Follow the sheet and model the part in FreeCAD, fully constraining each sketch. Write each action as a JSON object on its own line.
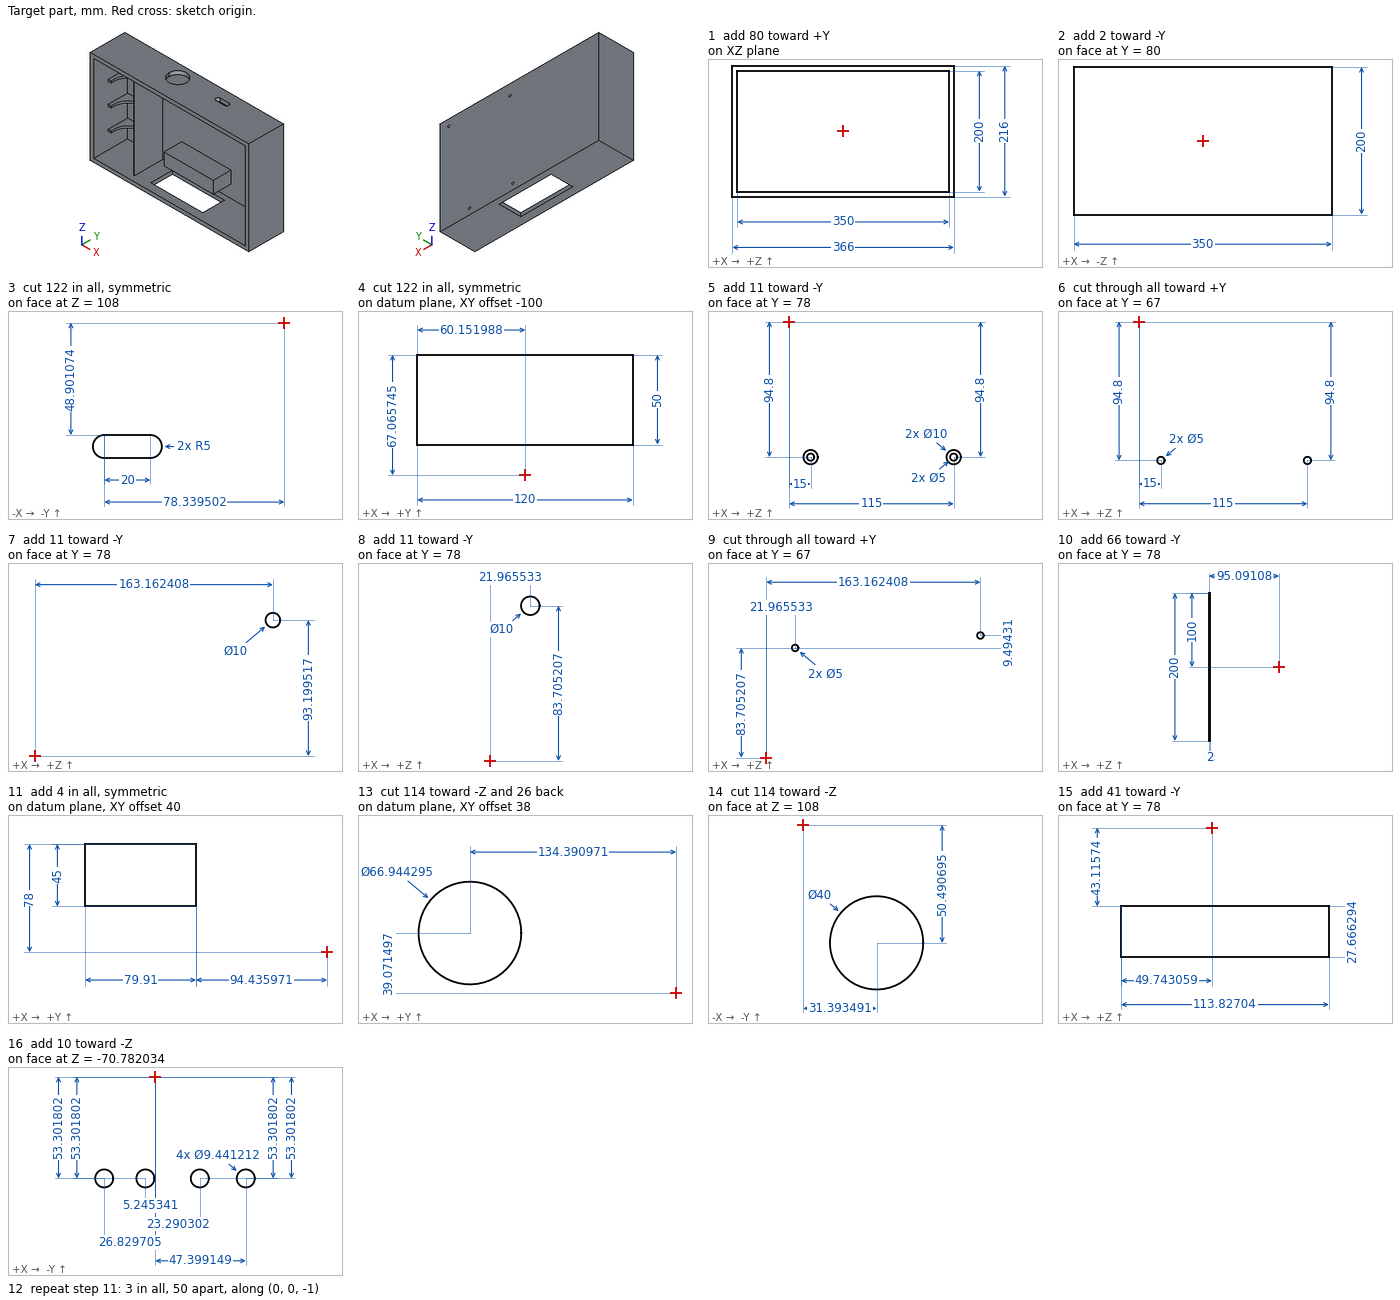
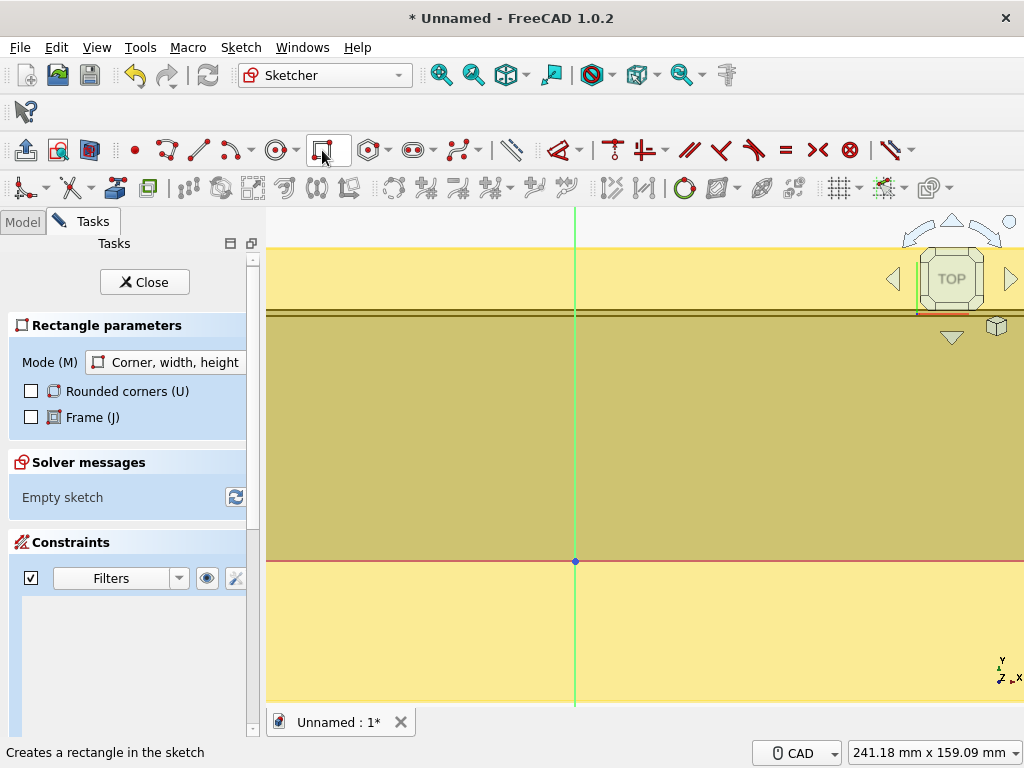
{"action": "left_click", "coordinate": [386, 350]}
{"action": "mouse_move", "coordinate": [763, 508]}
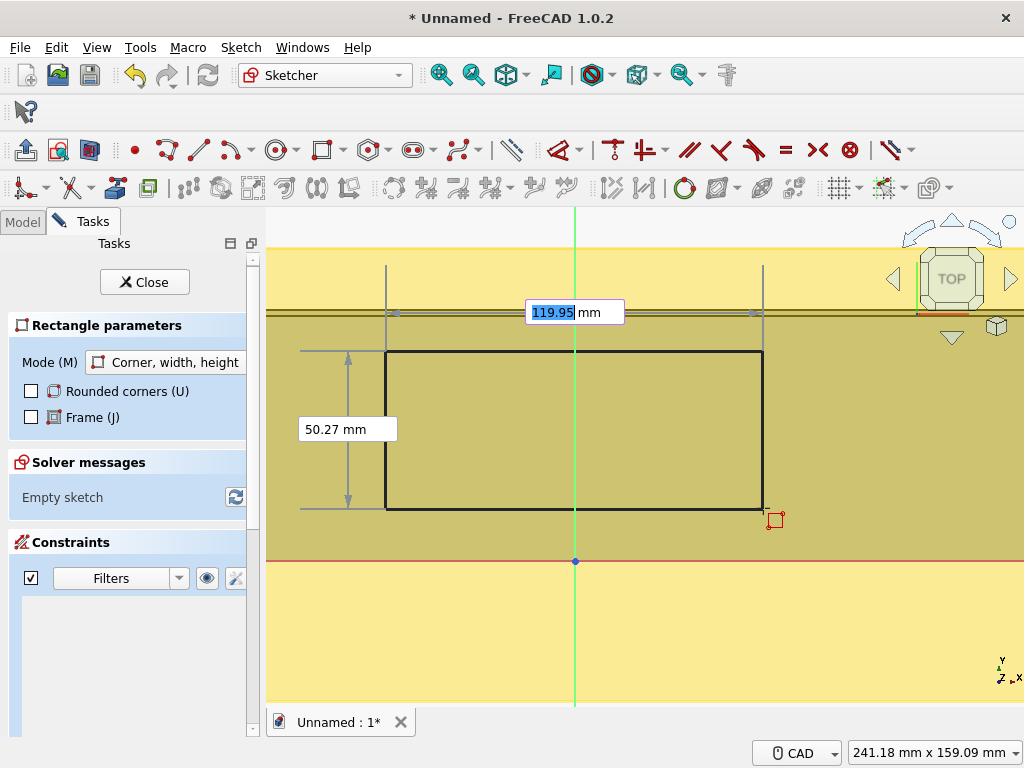
{"action": "type", "text": "120"}
{"action": "key", "text": "Tab"}
{"action": "type", "text": "50"}
{"action": "key", "text": "Return"}
{"action": "key", "text": "Escape"}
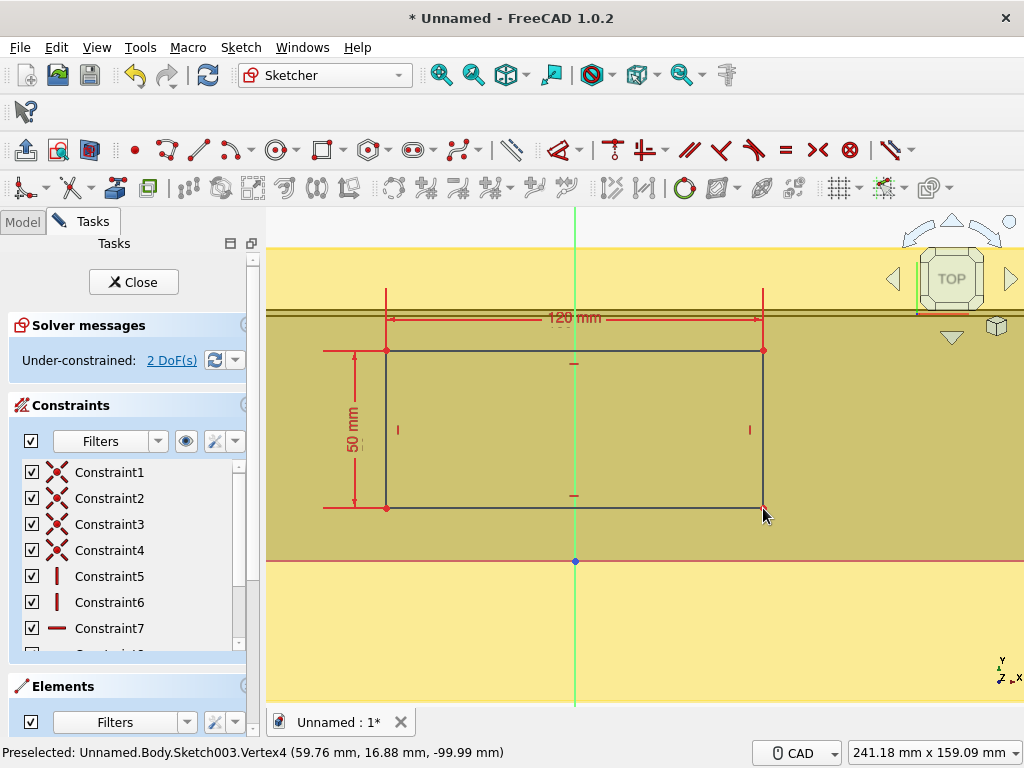
{"action": "left_click", "coordinate": [558, 150]}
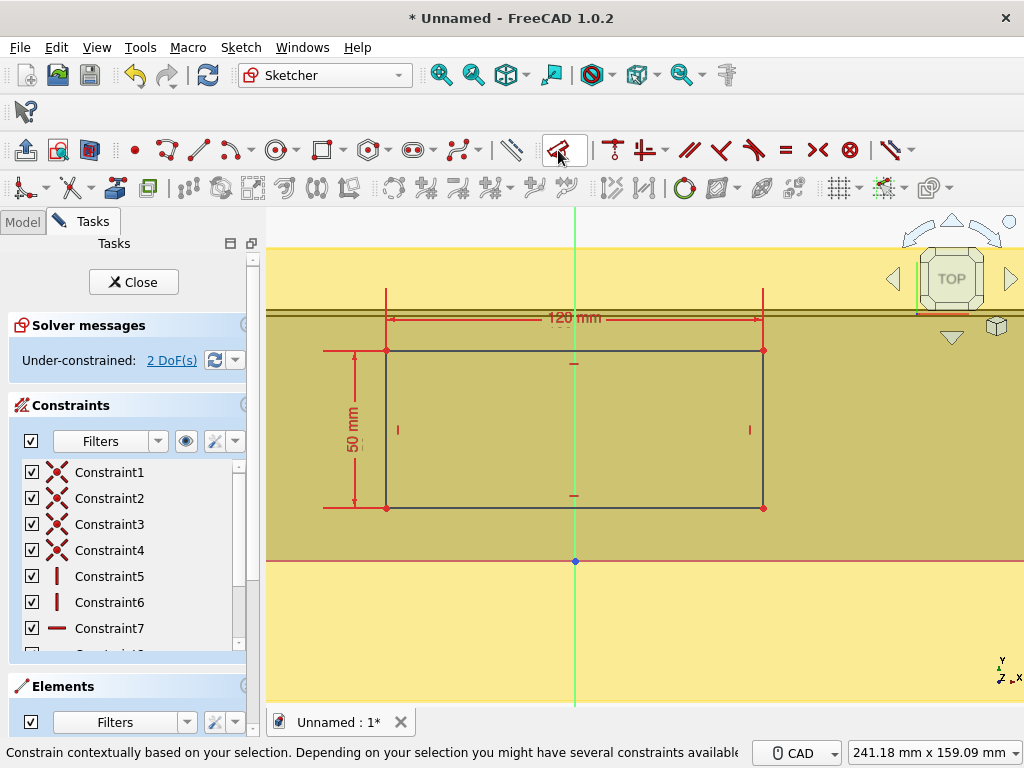
{"action": "left_click", "coordinate": [386, 351]}
{"action": "left_click", "coordinate": [481, 595]}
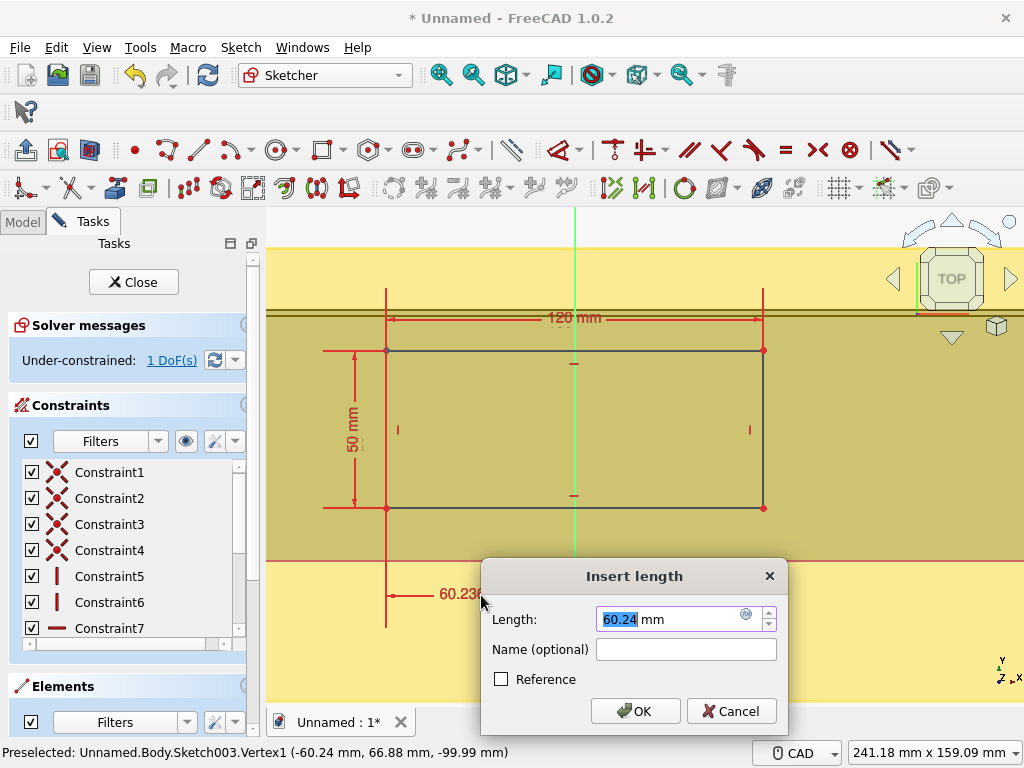
{"action": "type", "text": "60.151988"}
{"action": "key", "text": "Return"}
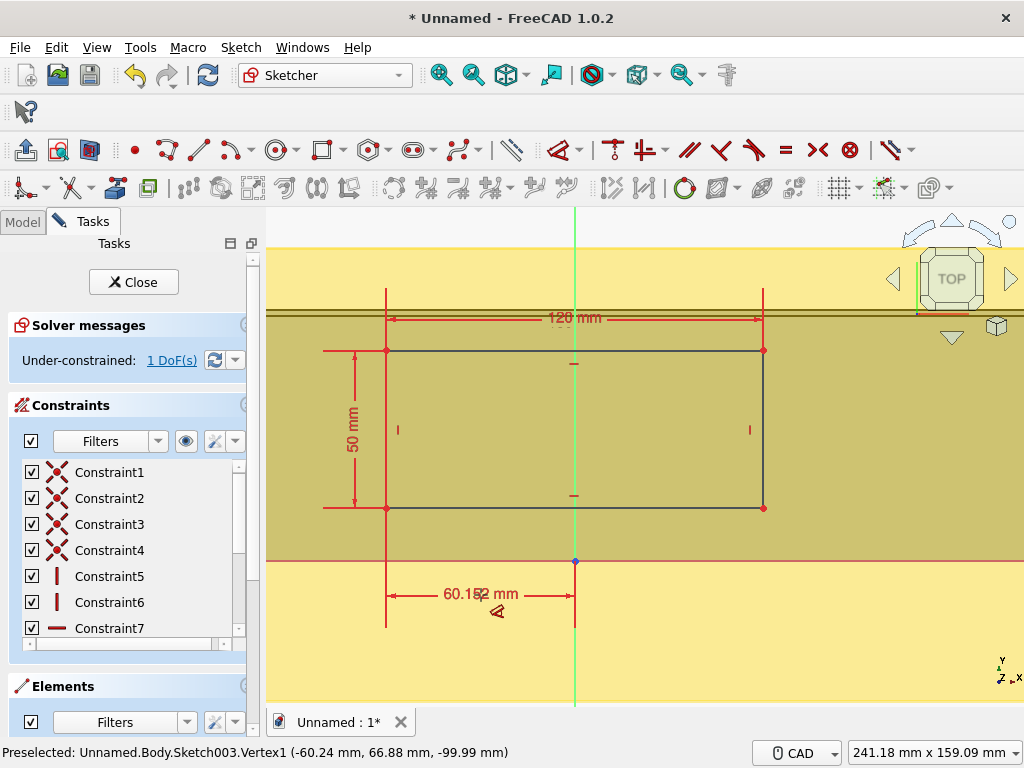
{"action": "left_click", "coordinate": [386, 351]}
{"action": "left_click", "coordinate": [352, 456]}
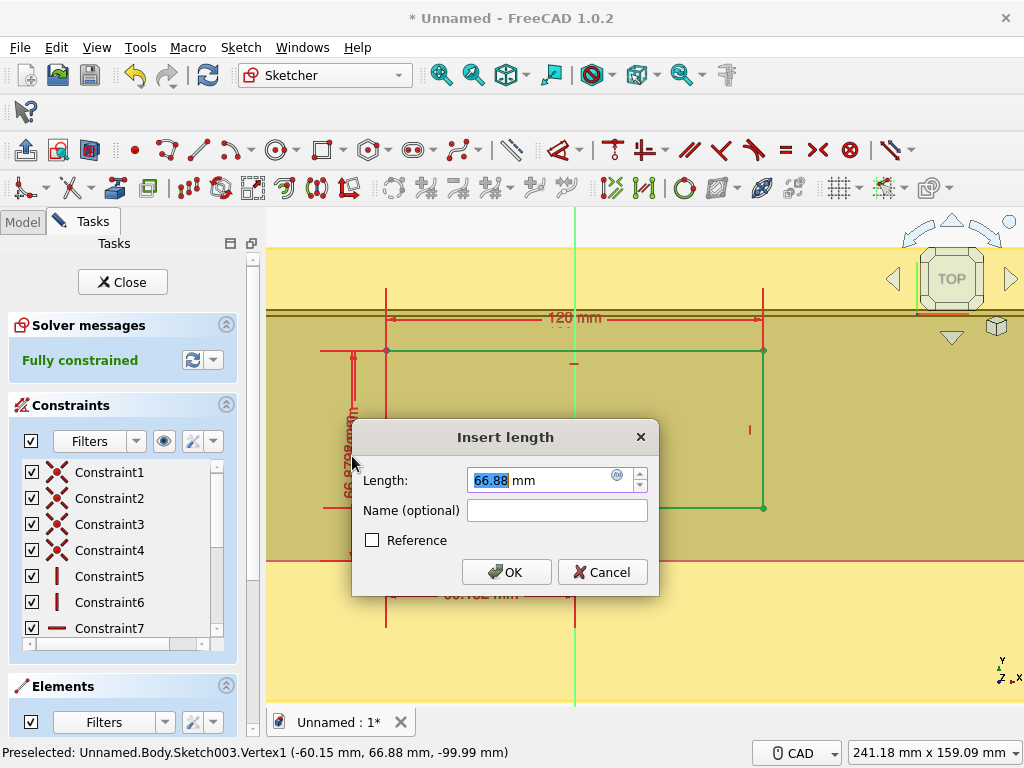
{"action": "type", "text": "67.065745"}
{"action": "key", "text": "Return"}
{"action": "key", "text": "Escape"}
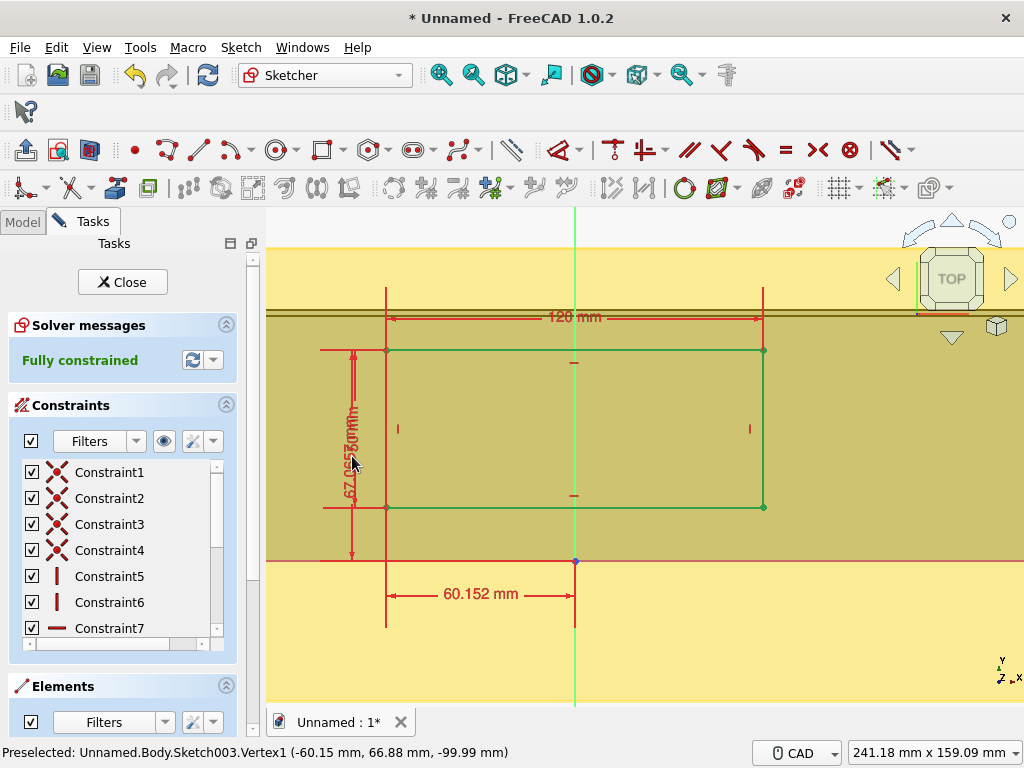
{"action": "left_click", "coordinate": [123, 282]}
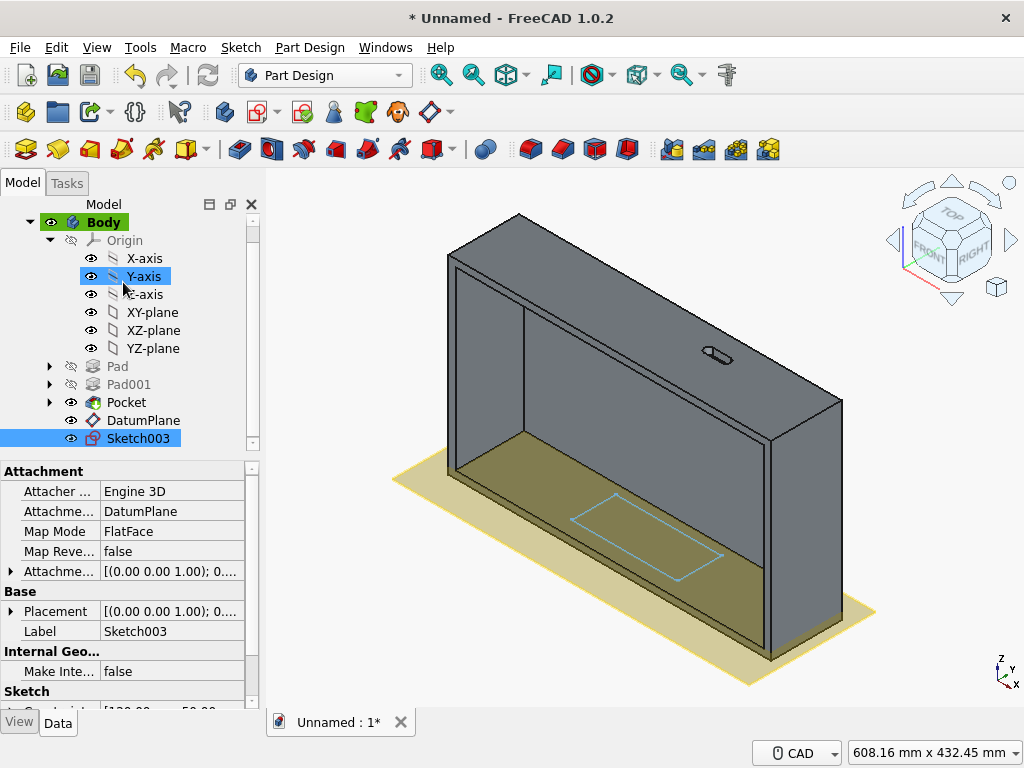
{"action": "left_click", "coordinate": [240, 150]}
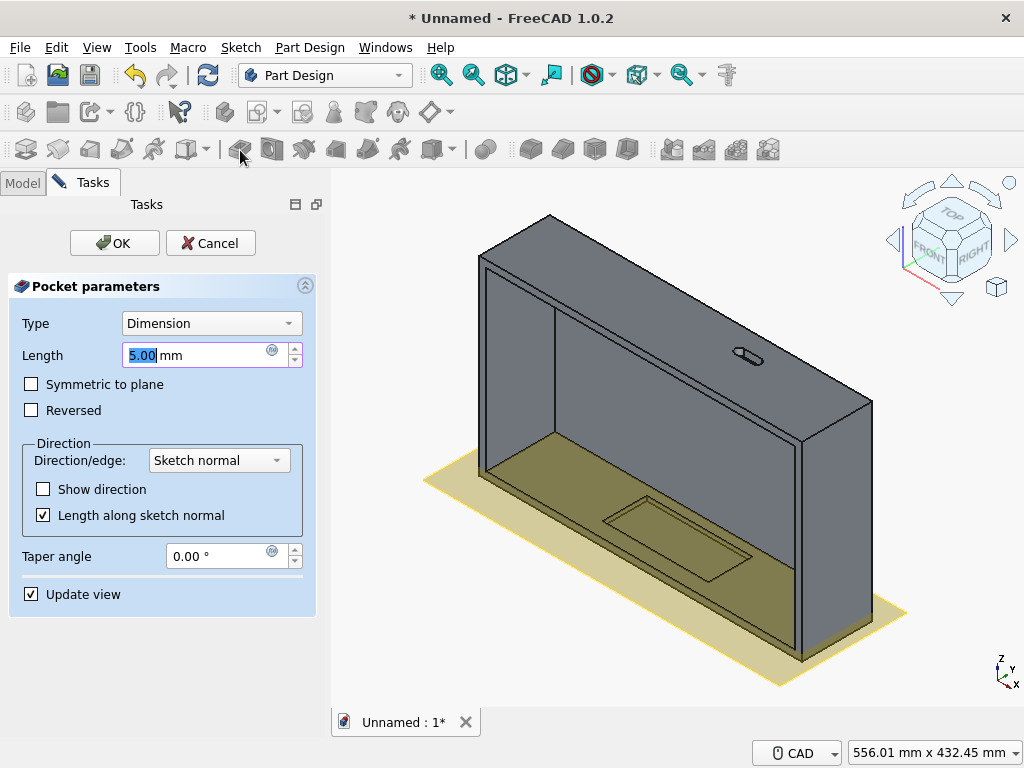
{"action": "type", "text": "122"}
{"action": "key", "text": "Tab"}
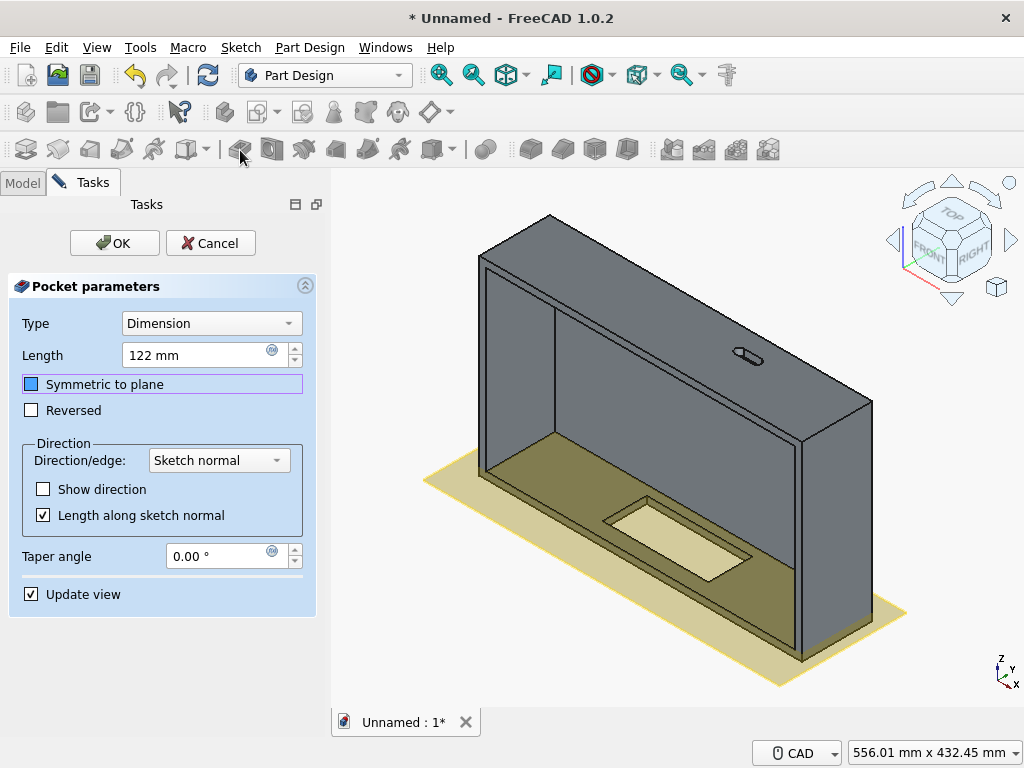
{"action": "left_click", "coordinate": [30, 384]}